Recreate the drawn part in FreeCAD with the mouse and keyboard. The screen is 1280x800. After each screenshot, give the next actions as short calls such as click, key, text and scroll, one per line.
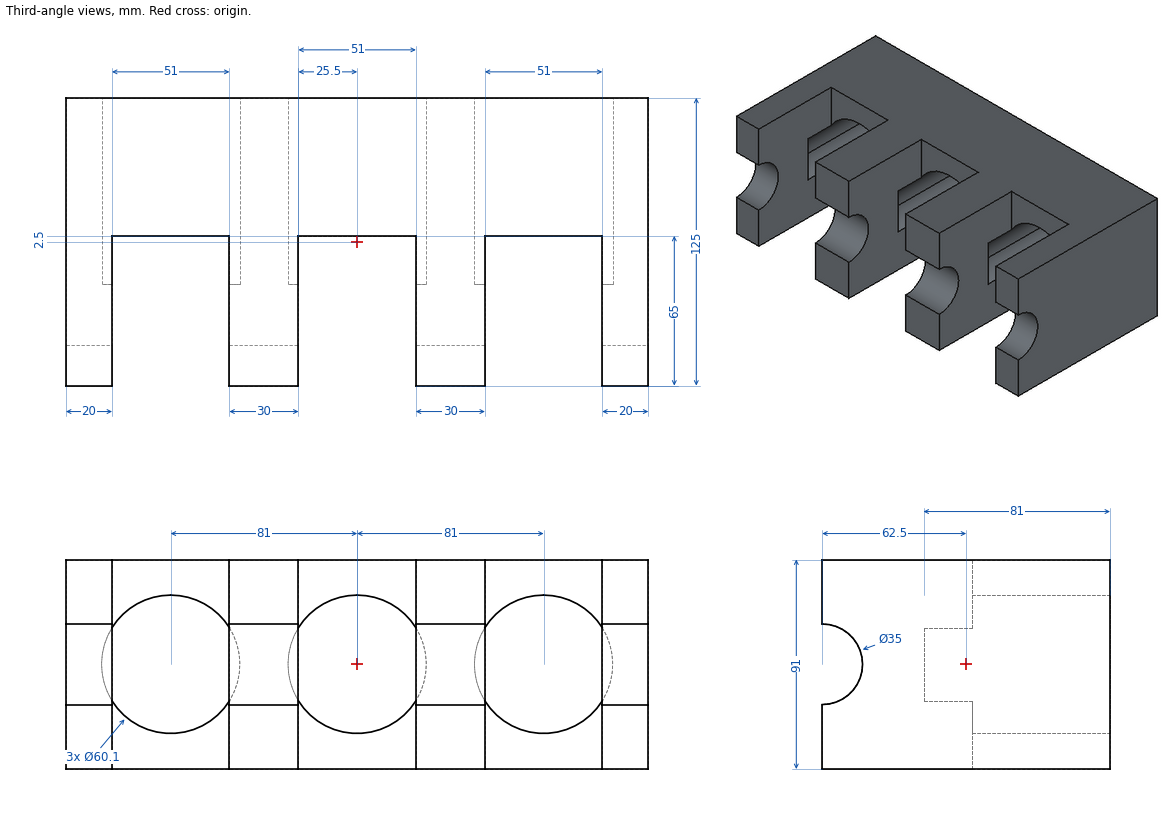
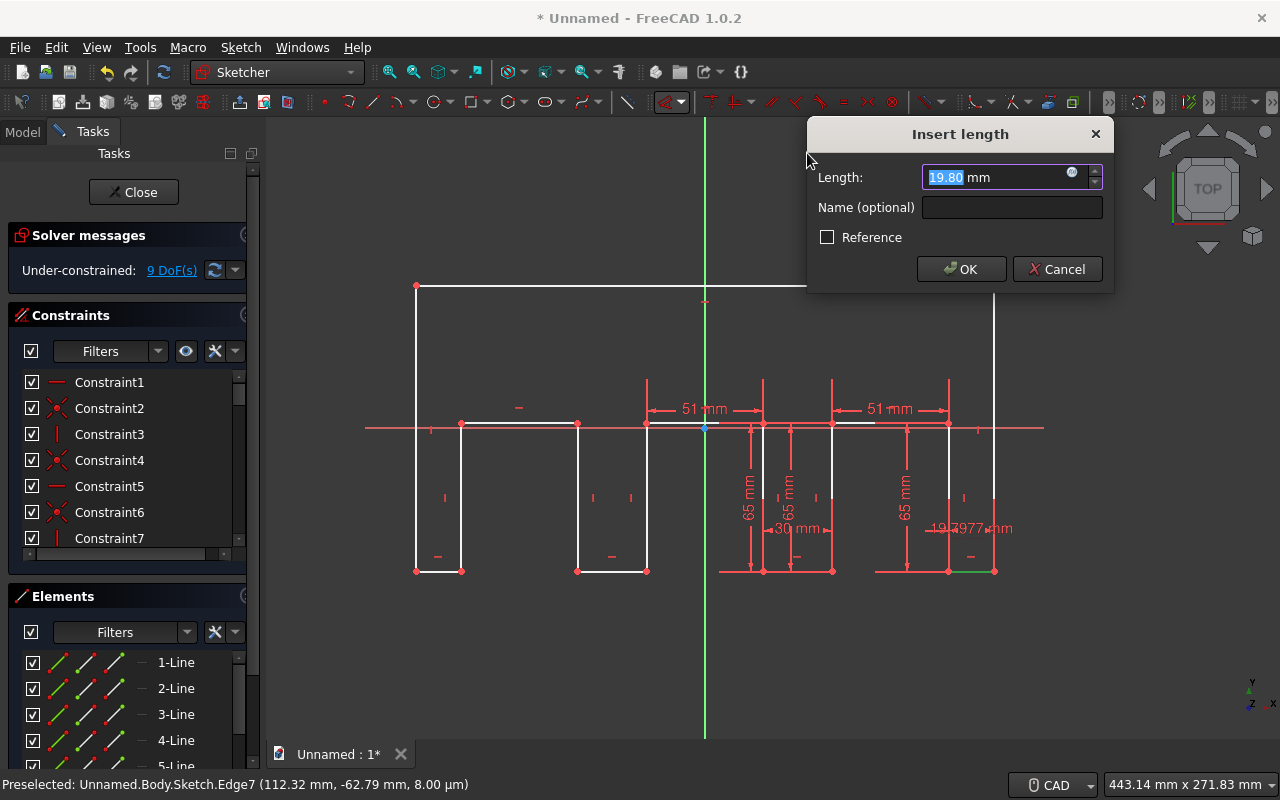
text(20)
key(Return)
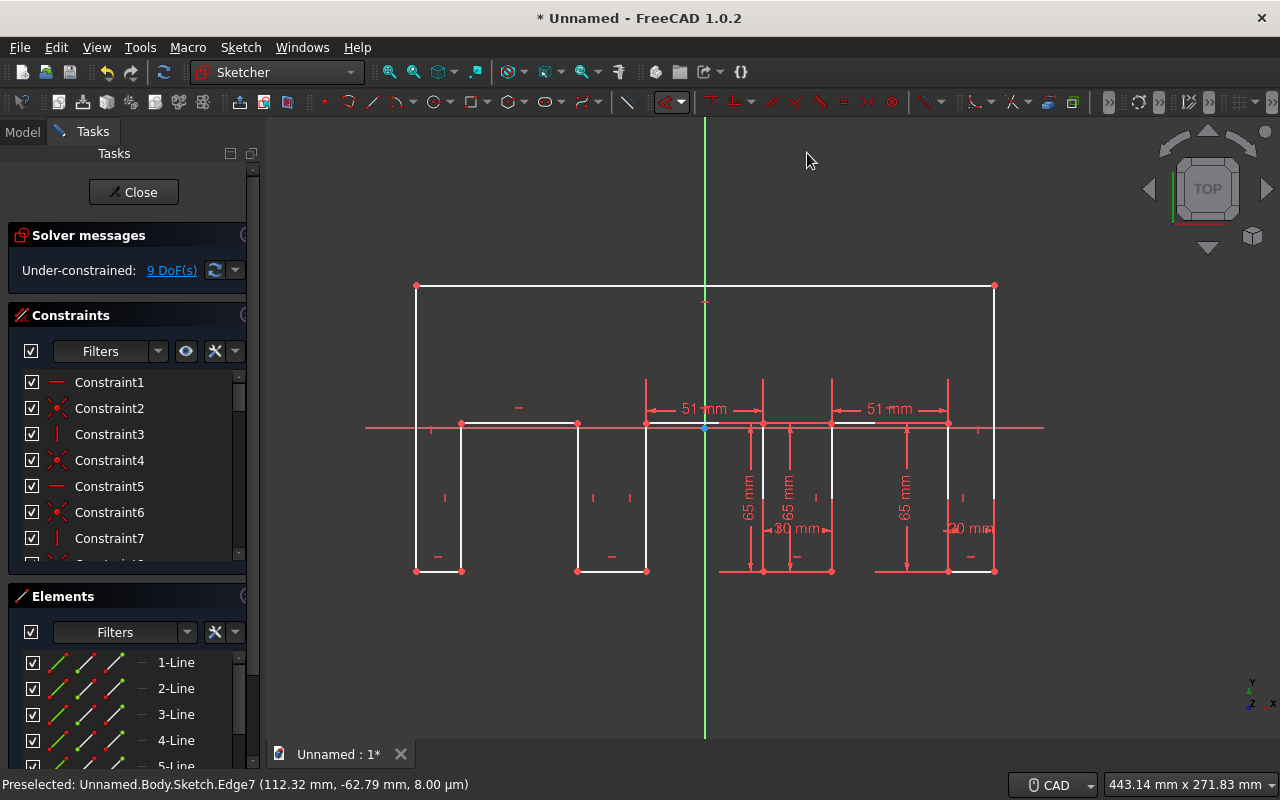
click(430, 572)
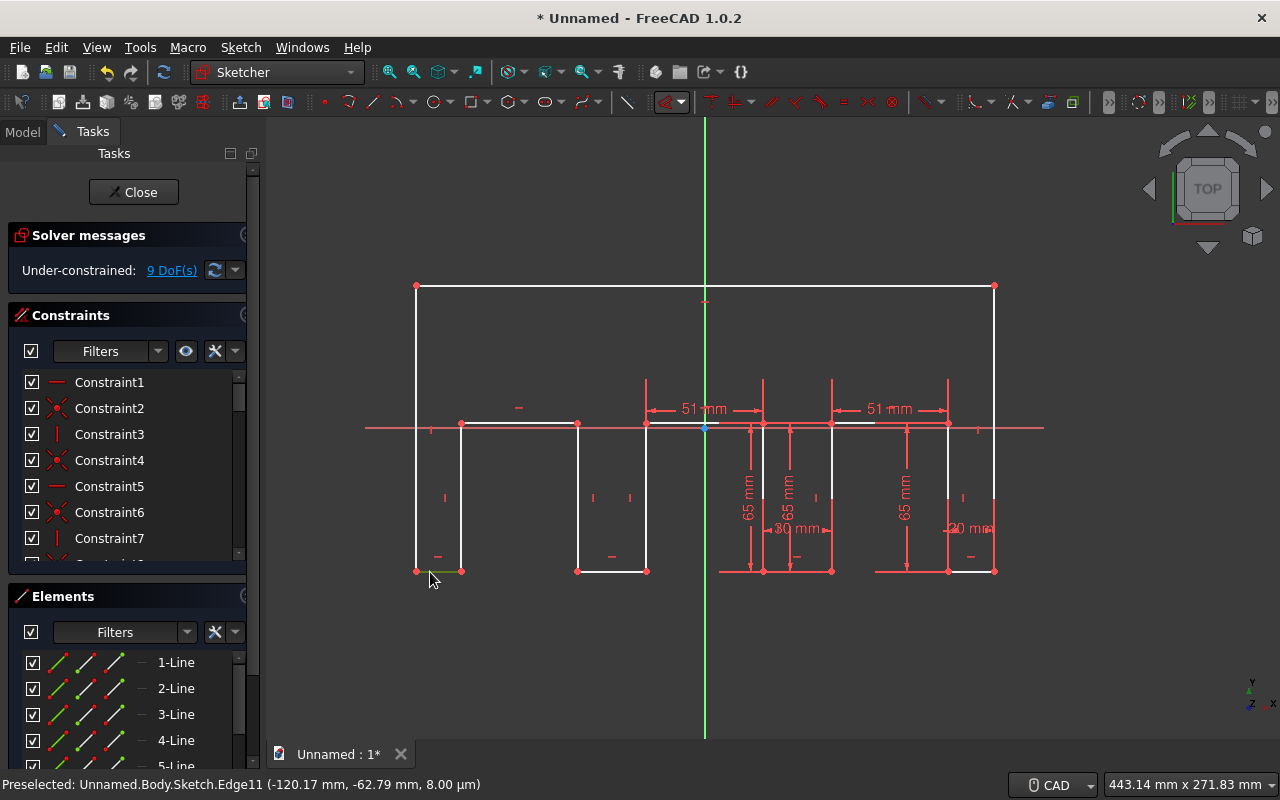
key(l)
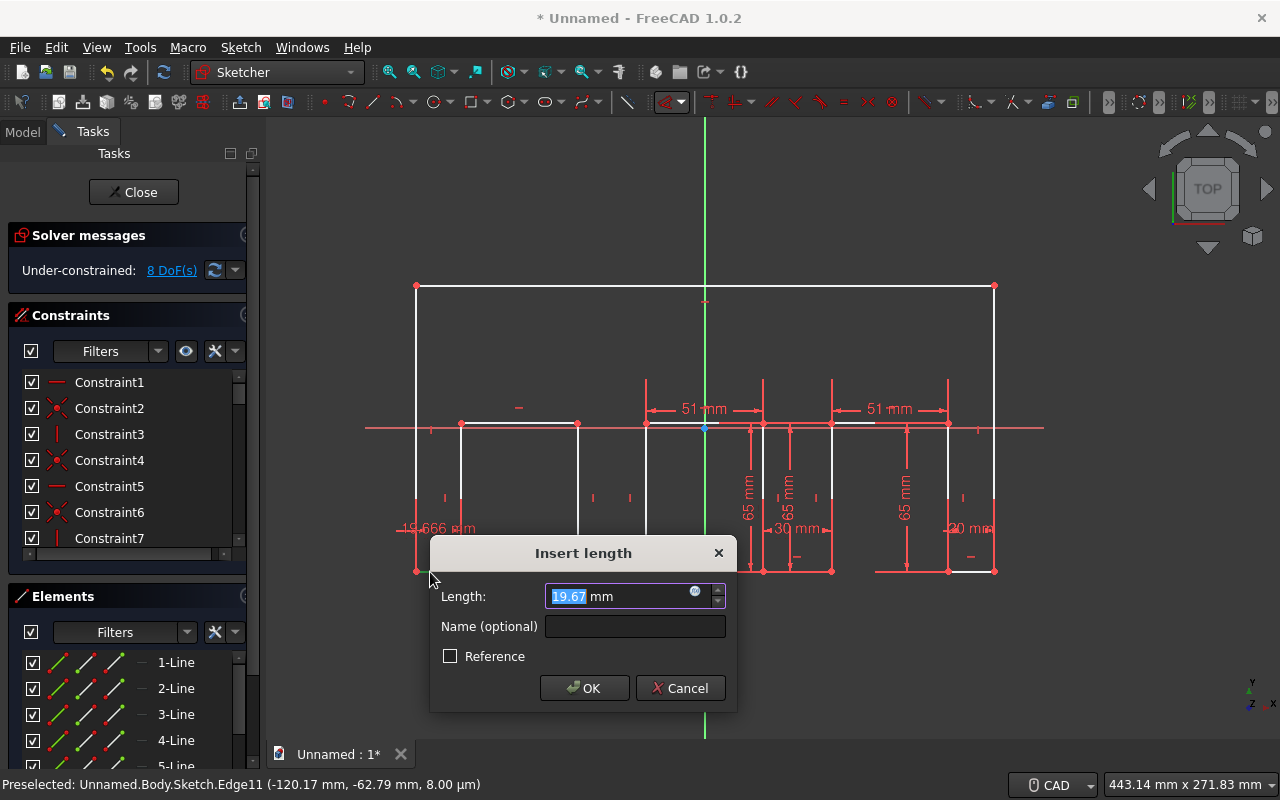
text(20)
key(Return)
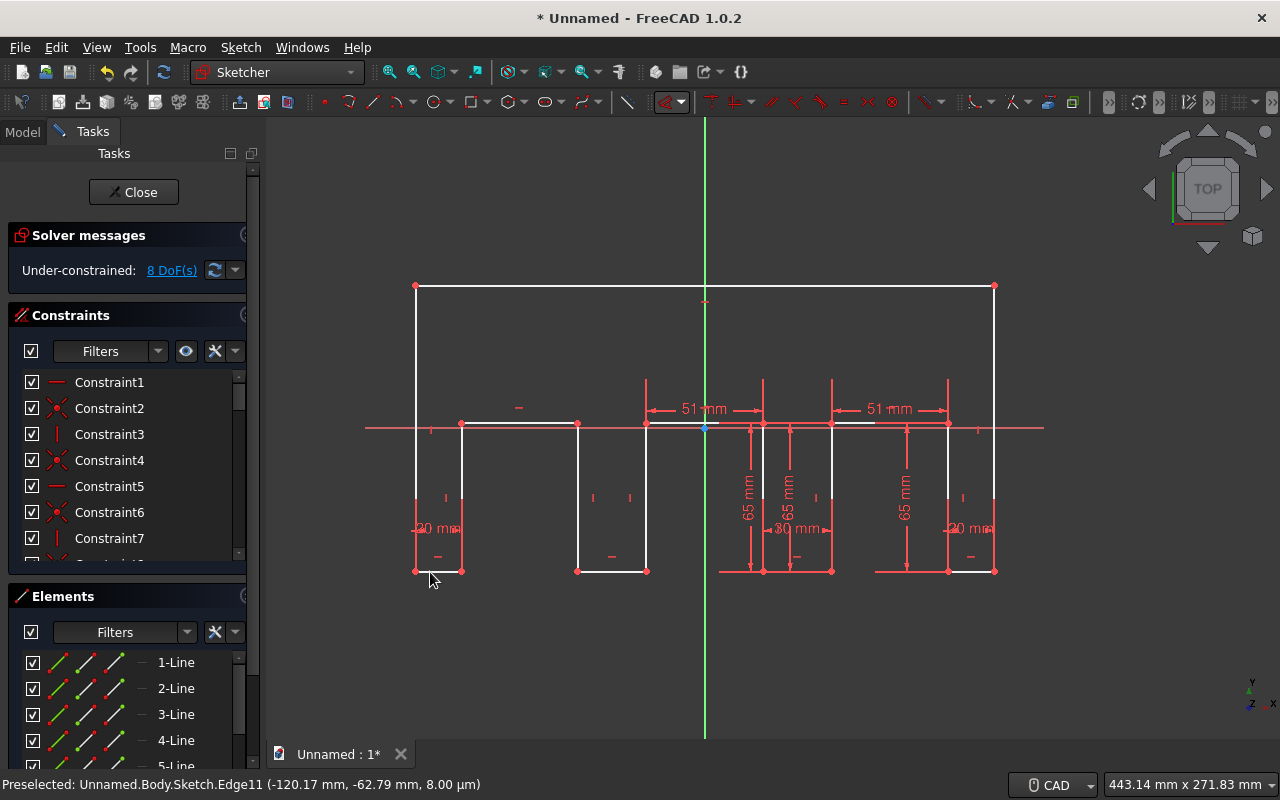
click(462, 527)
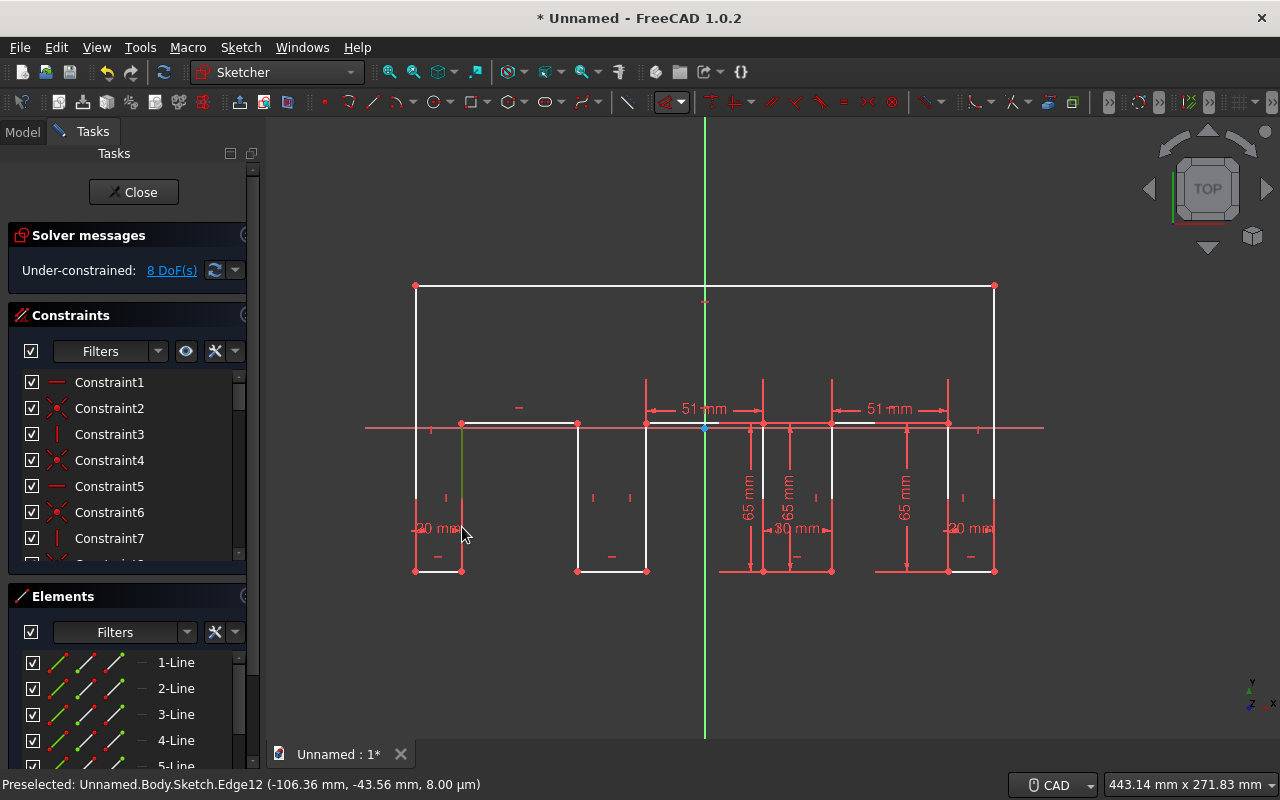
key(i)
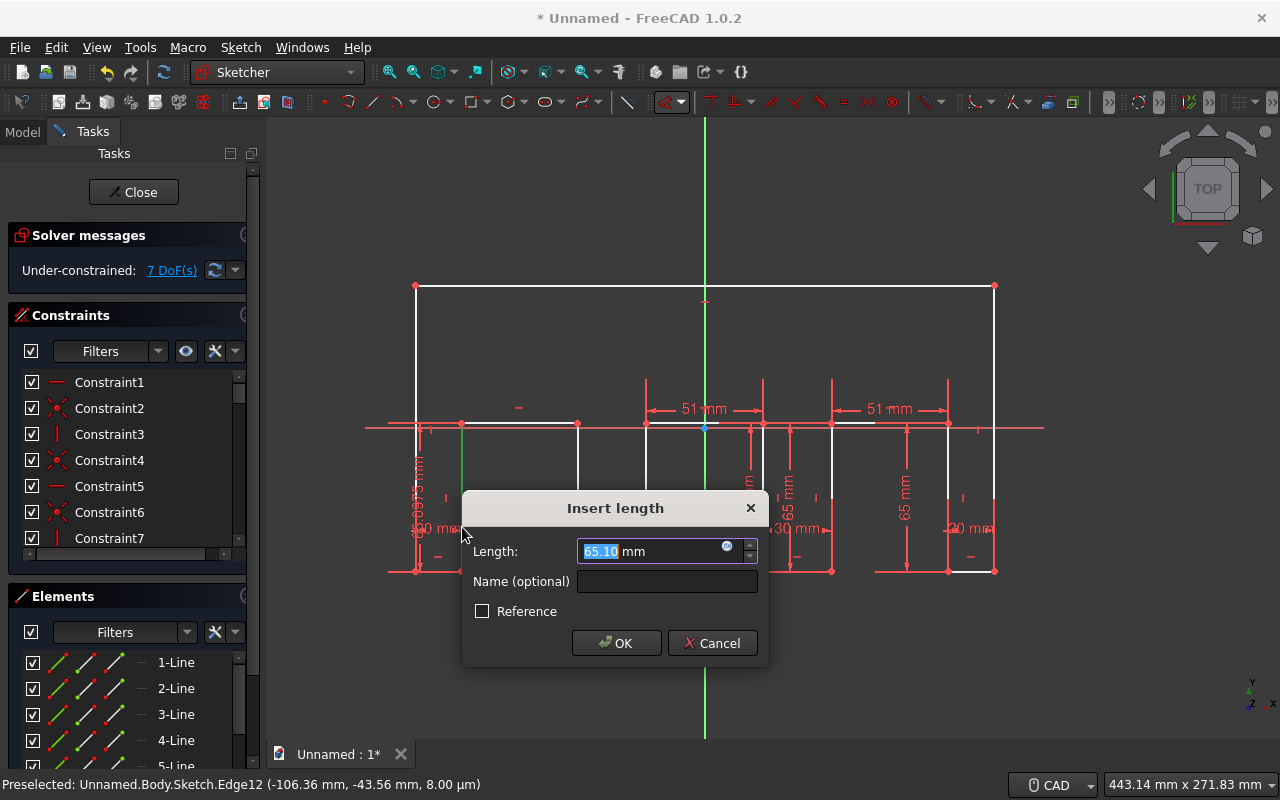
text(65)
key(Return)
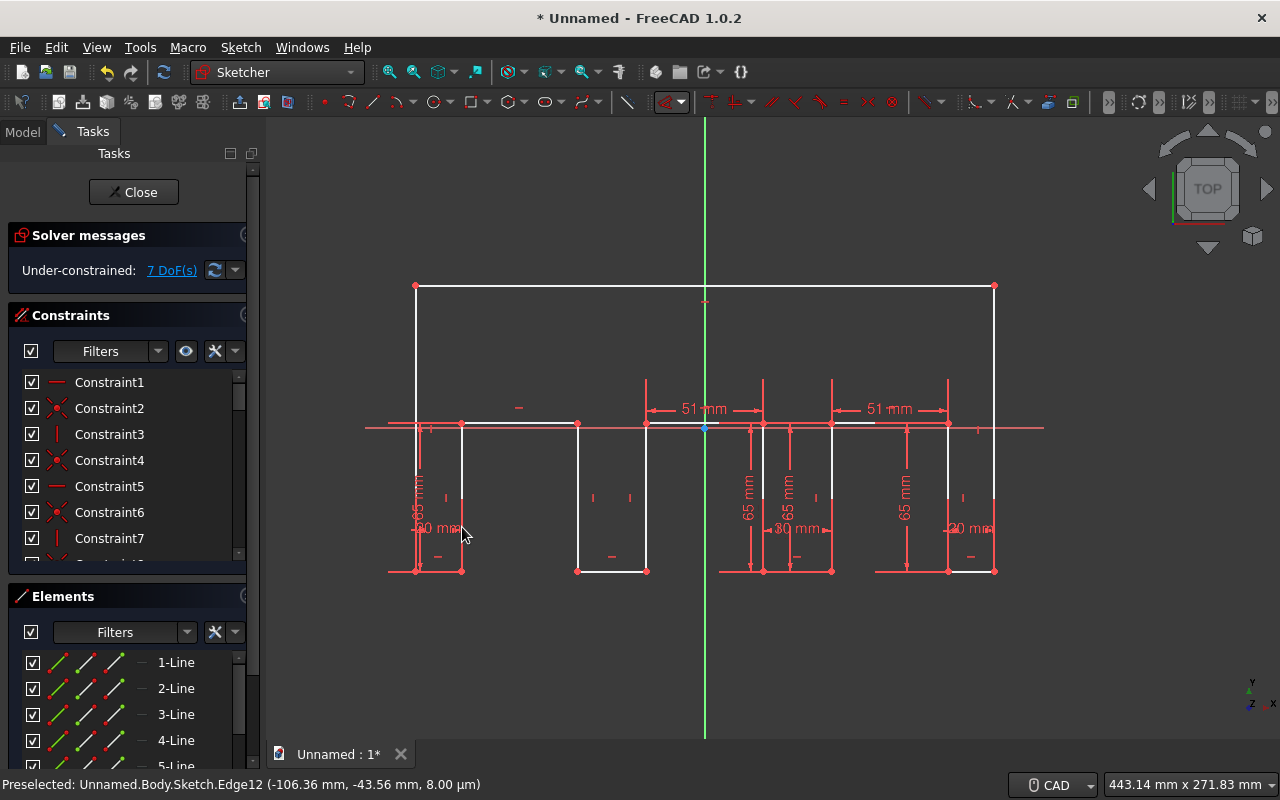
scroll(497, 423, up, 5)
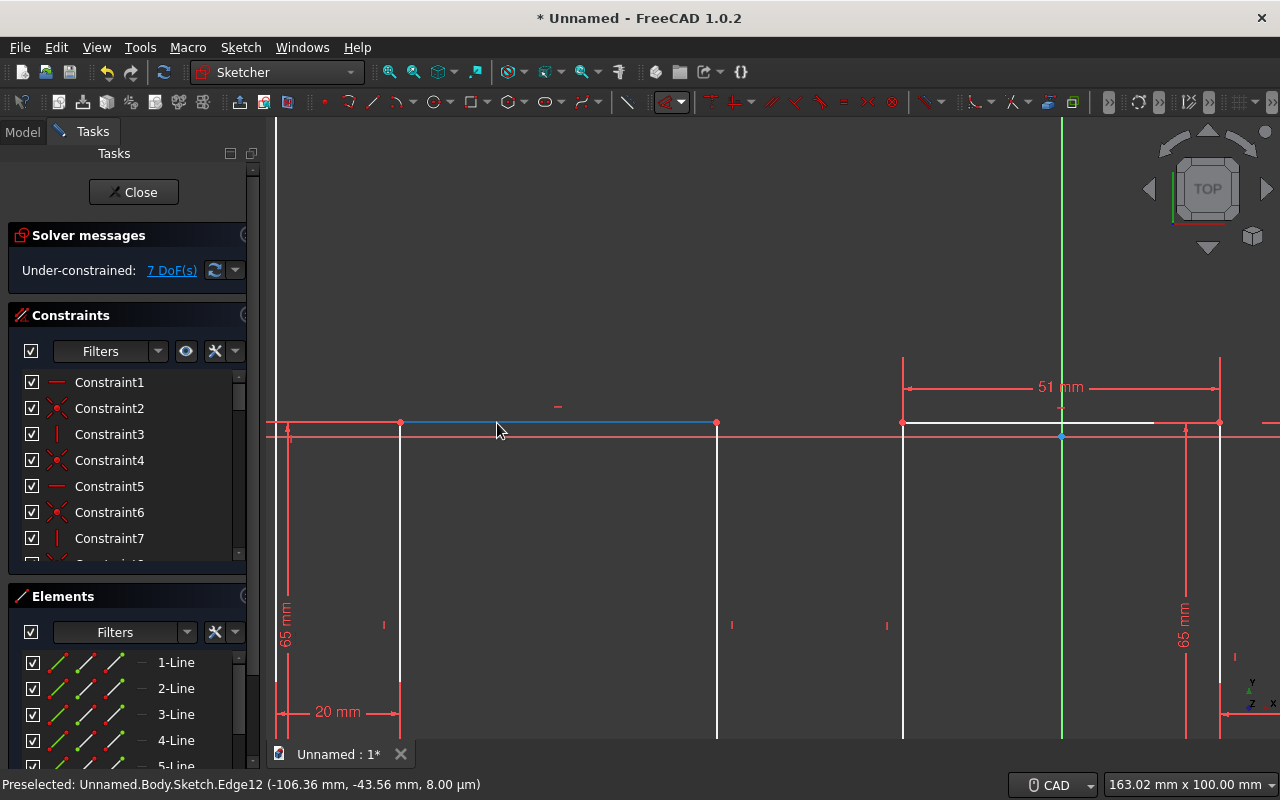
click(495, 422)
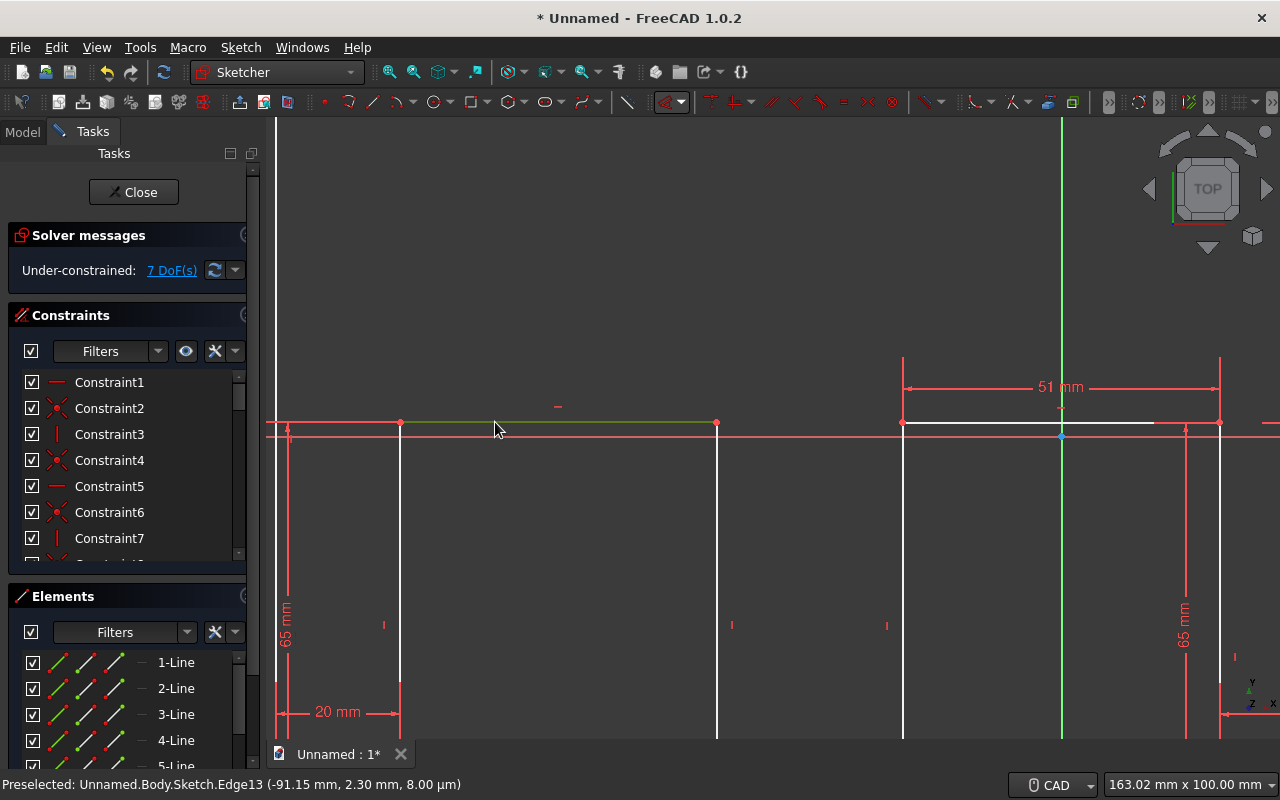
click(684, 102)